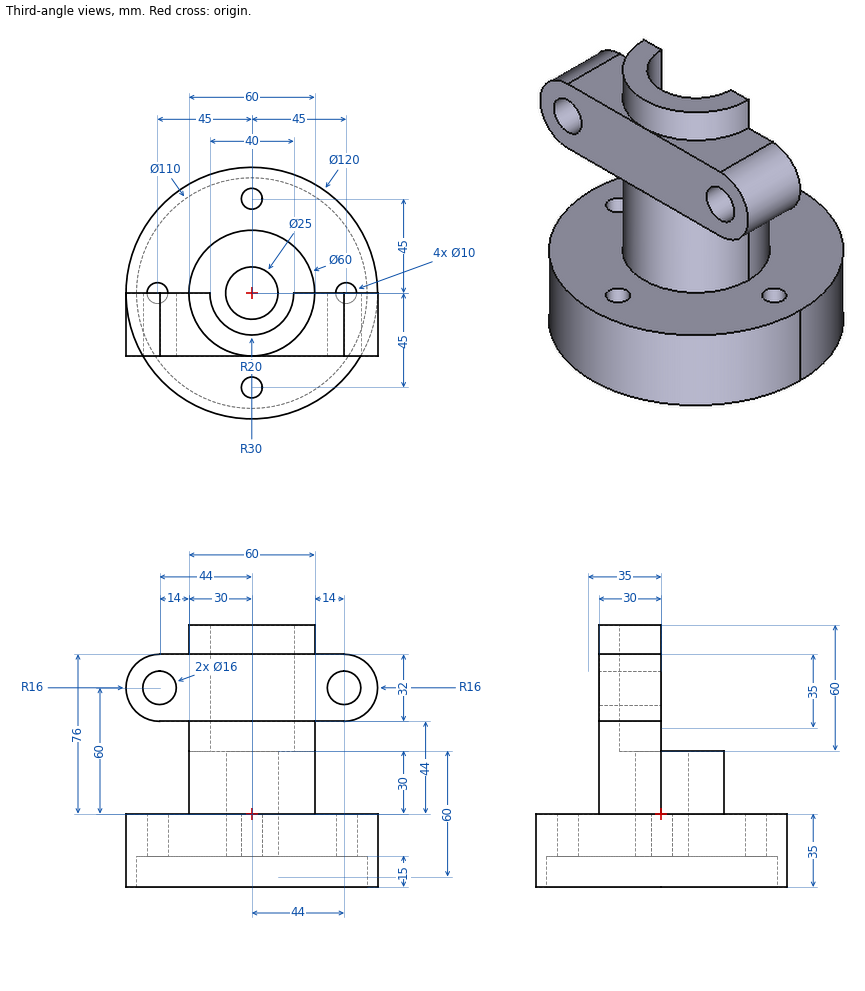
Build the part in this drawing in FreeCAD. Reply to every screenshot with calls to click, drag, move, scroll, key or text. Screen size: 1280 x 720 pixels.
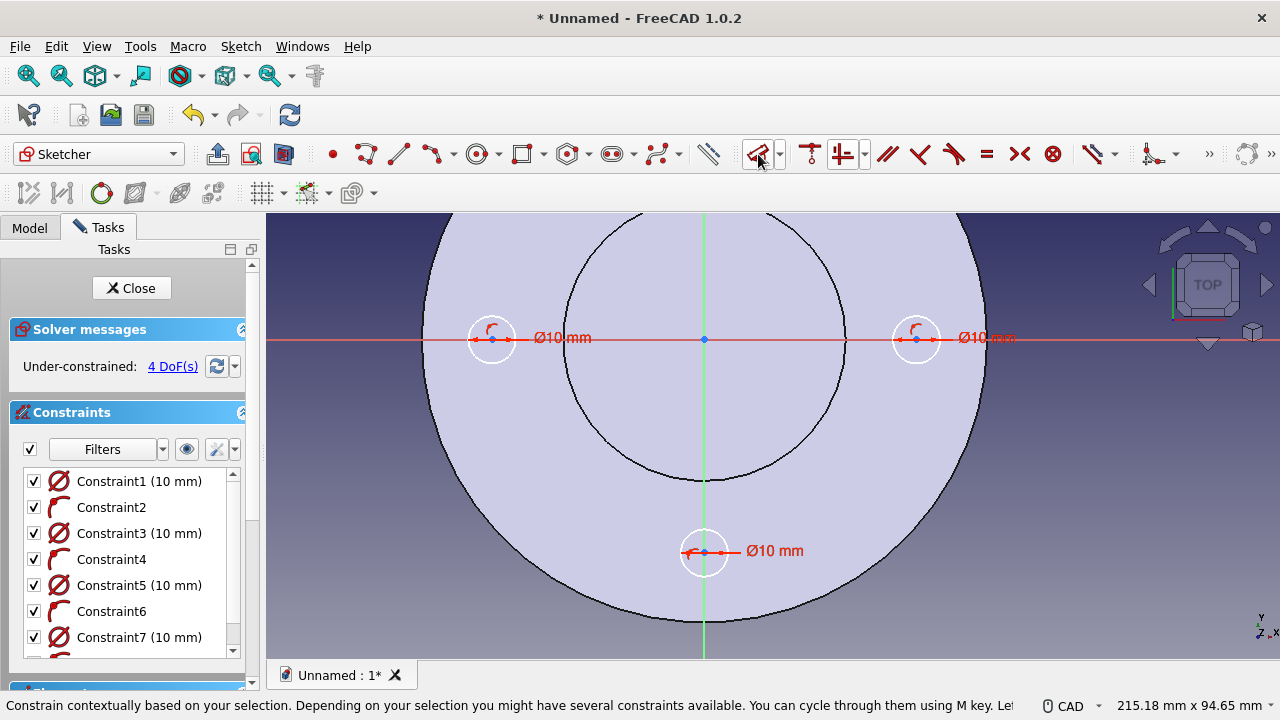
click(917, 340)
click(810, 374)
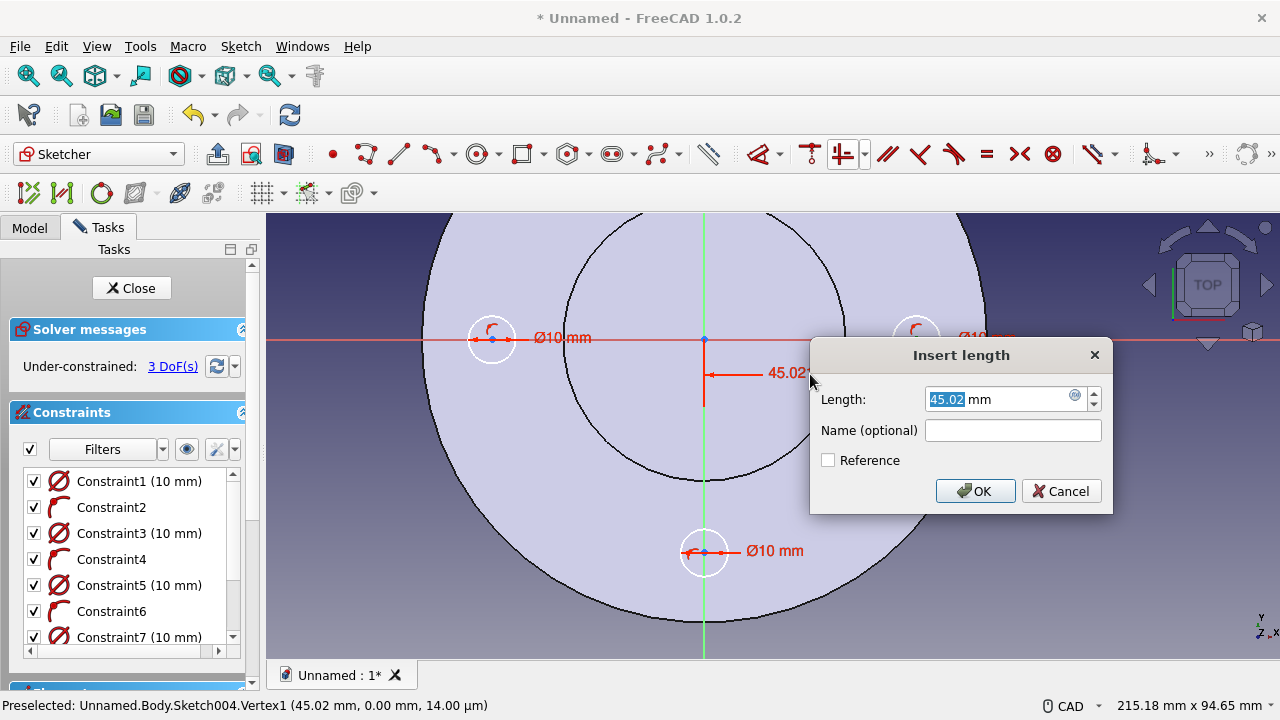
text(45)
key(Return)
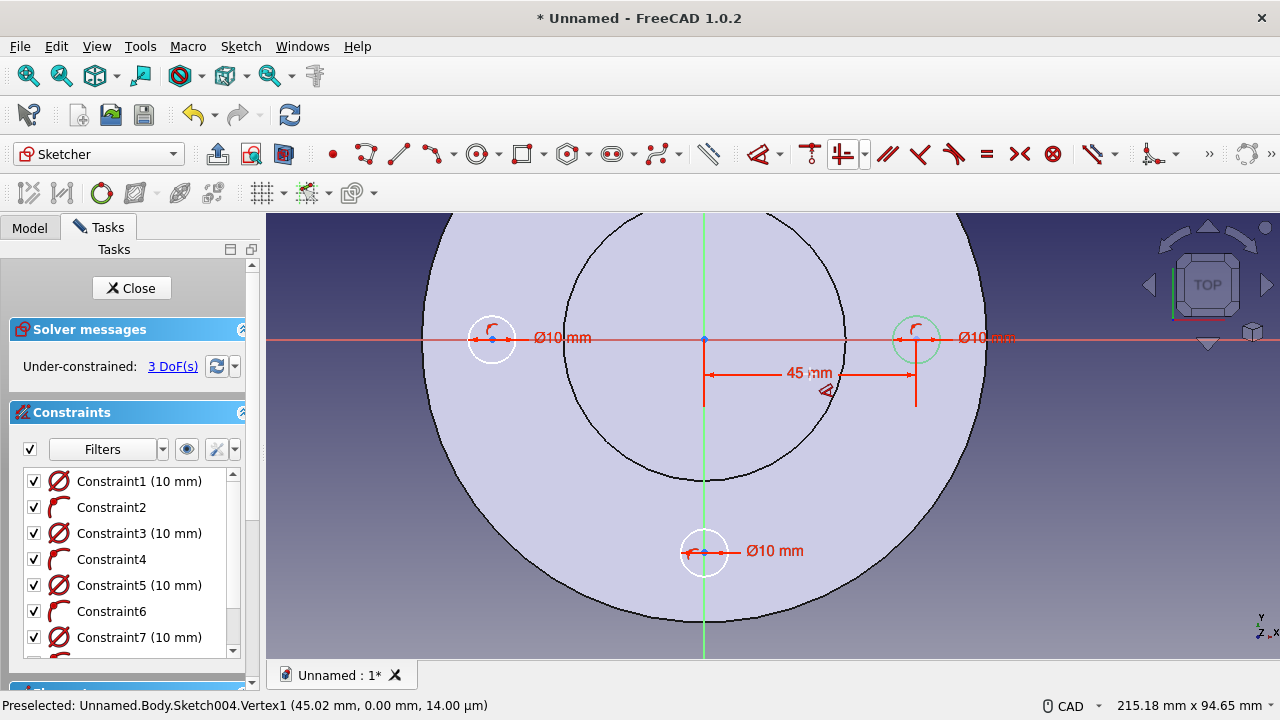
scroll(705, 553, down, 3)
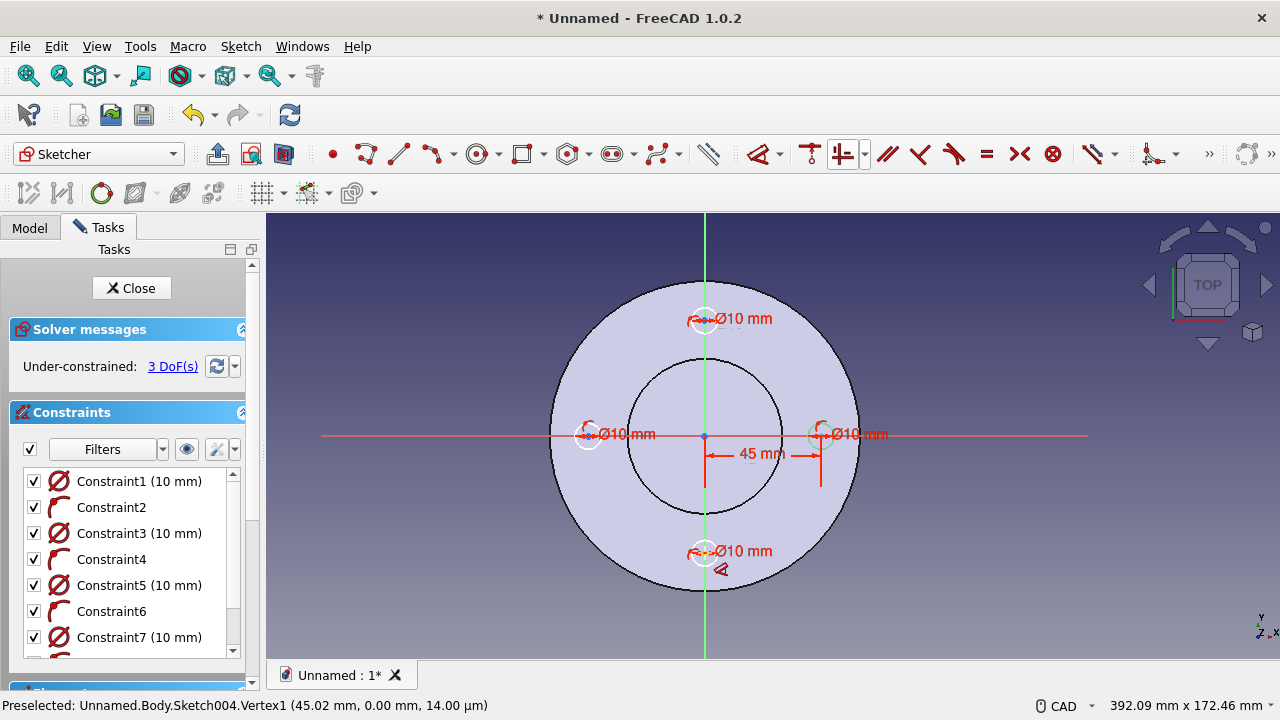
click(705, 321)
click(739, 378)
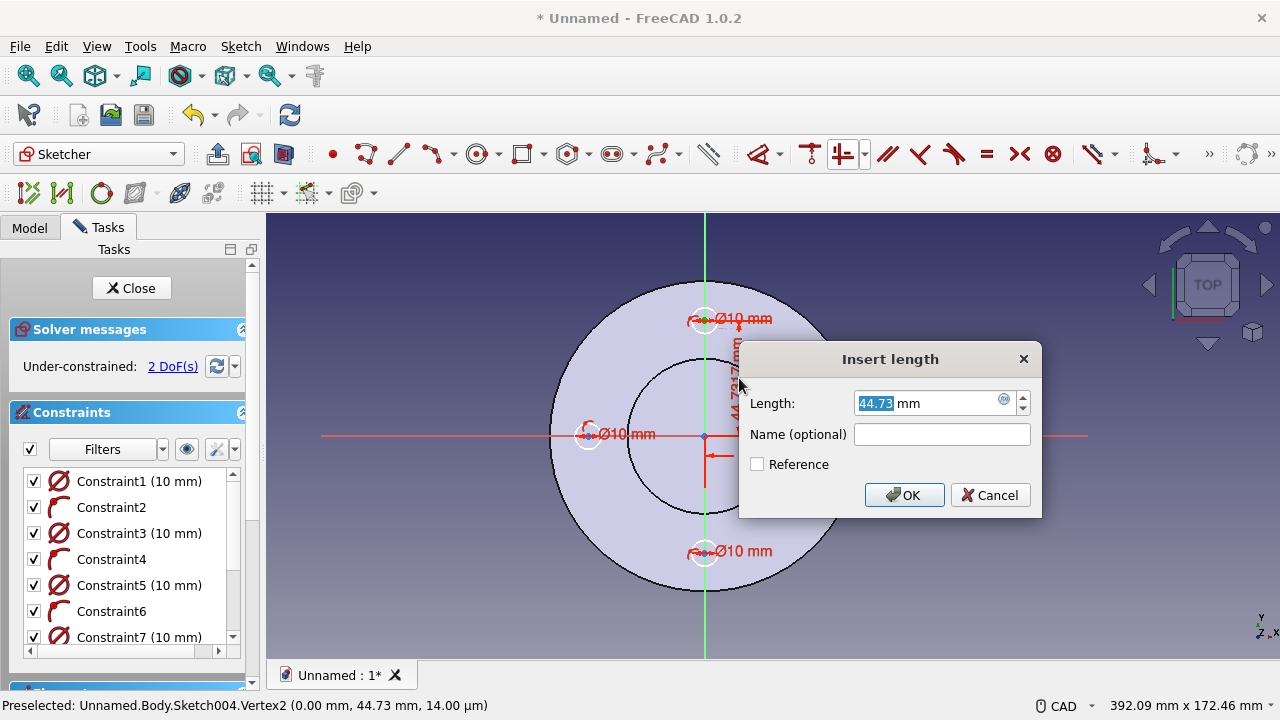
text(45)
key(Return)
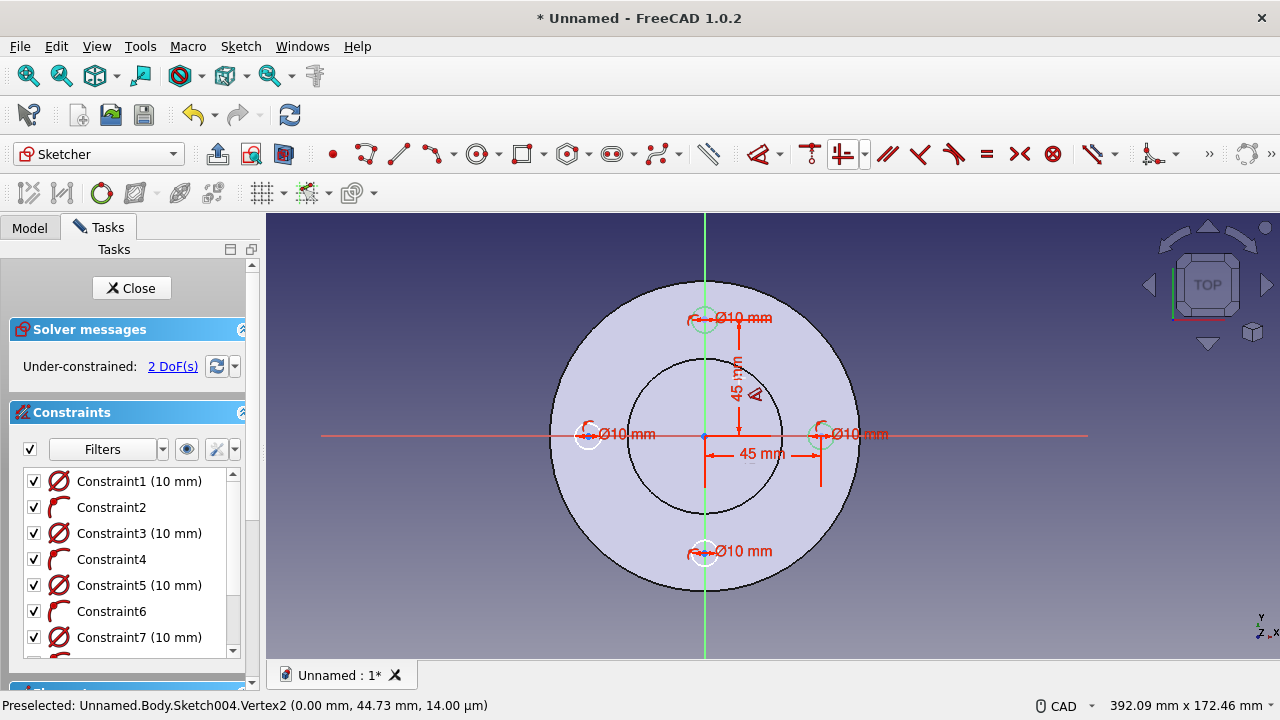
click(588, 436)
click(647, 470)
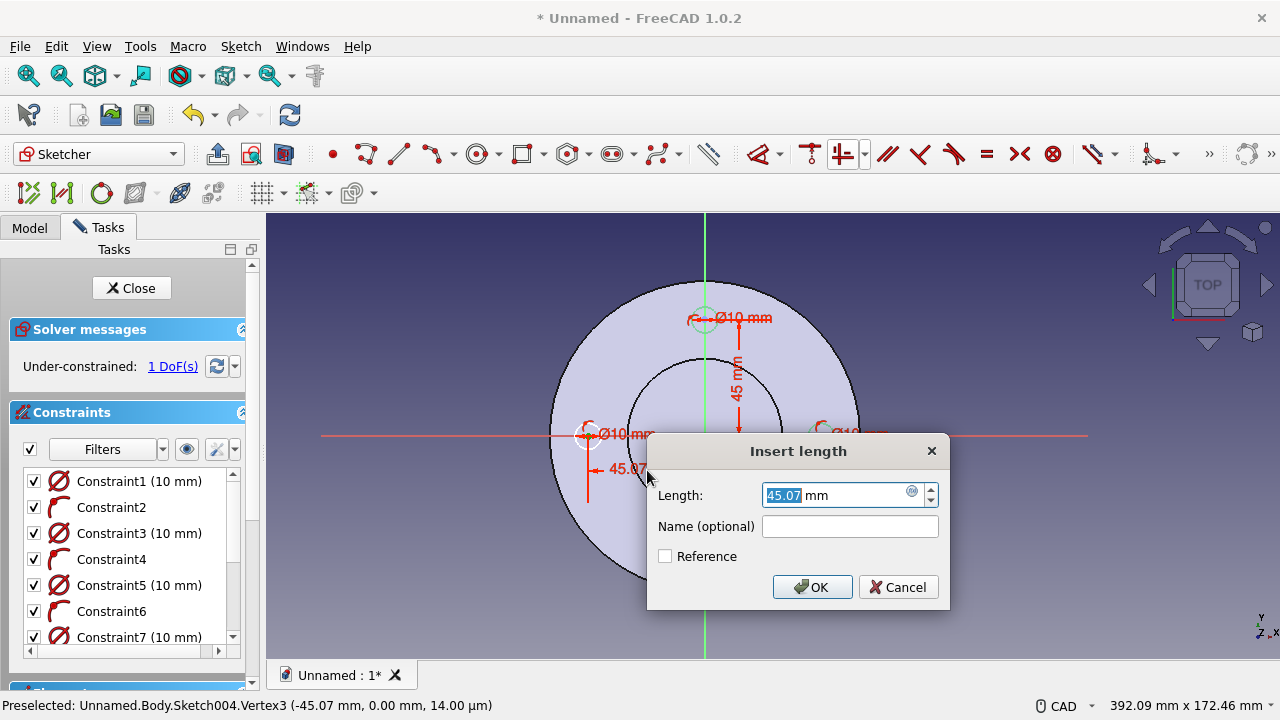
text(45)
key(Return)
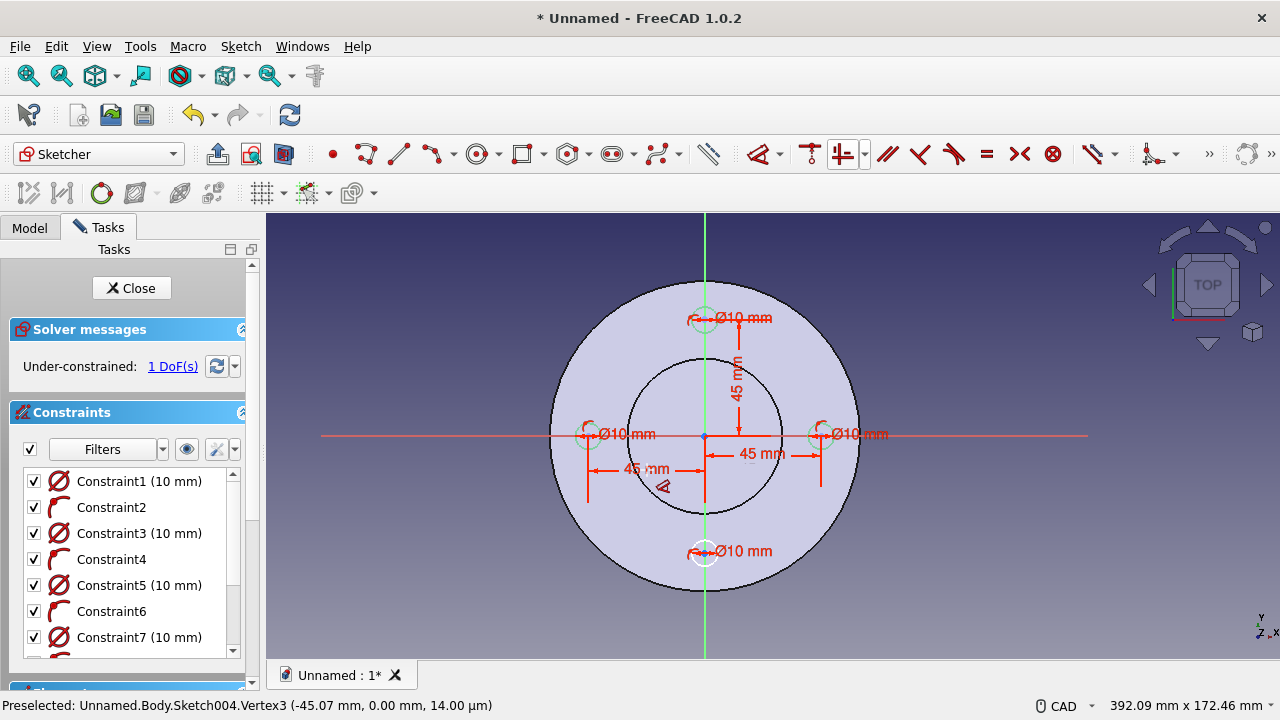
click(705, 553)
click(739, 495)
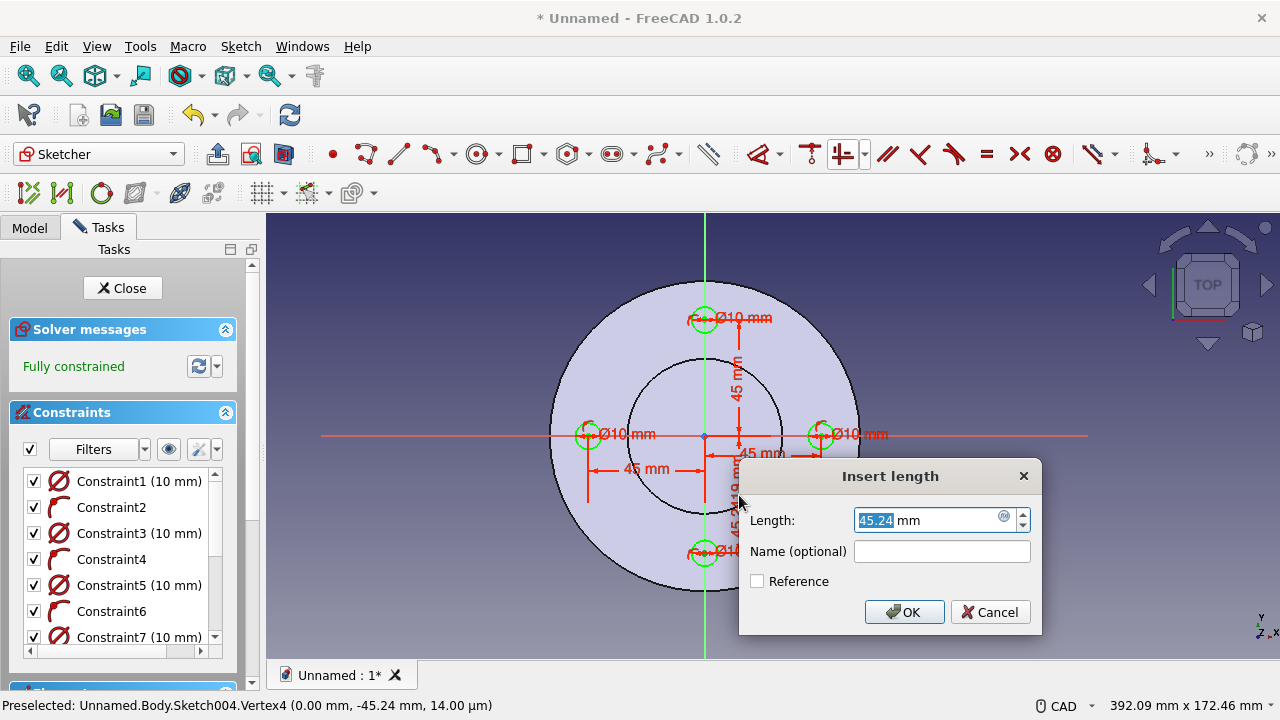
text(45)
key(Return)
key(Escape)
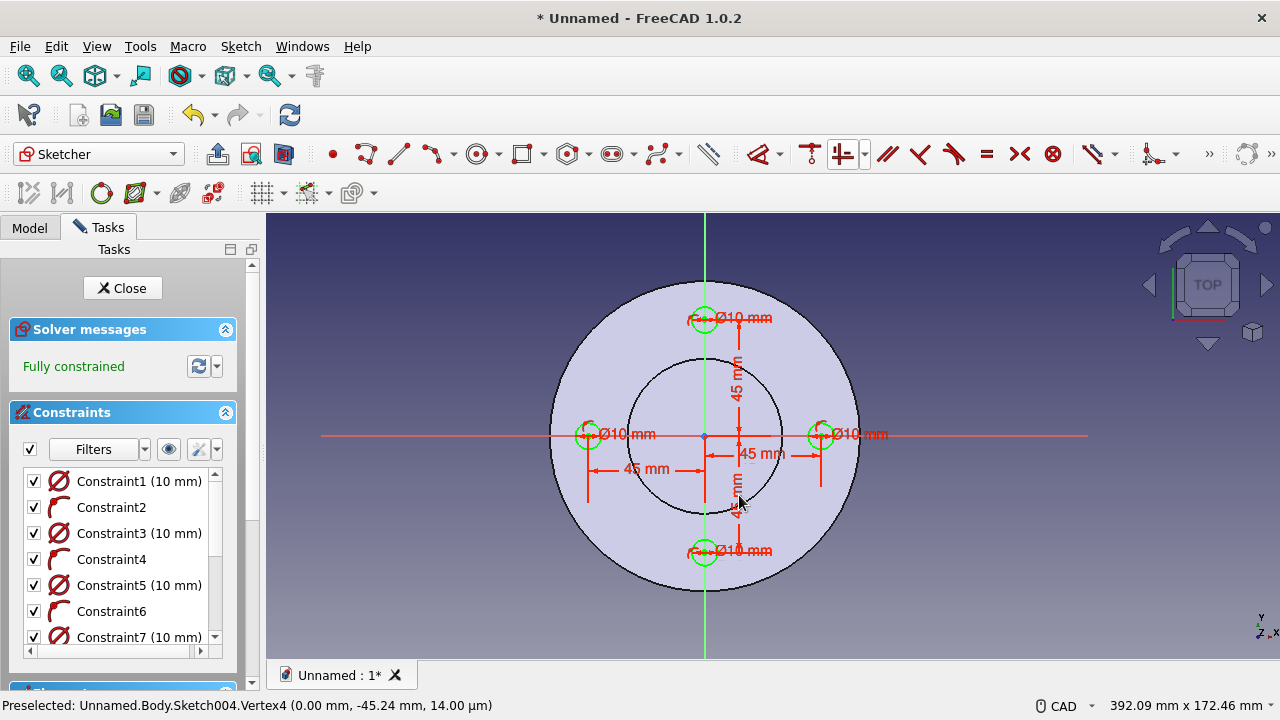
click(123, 288)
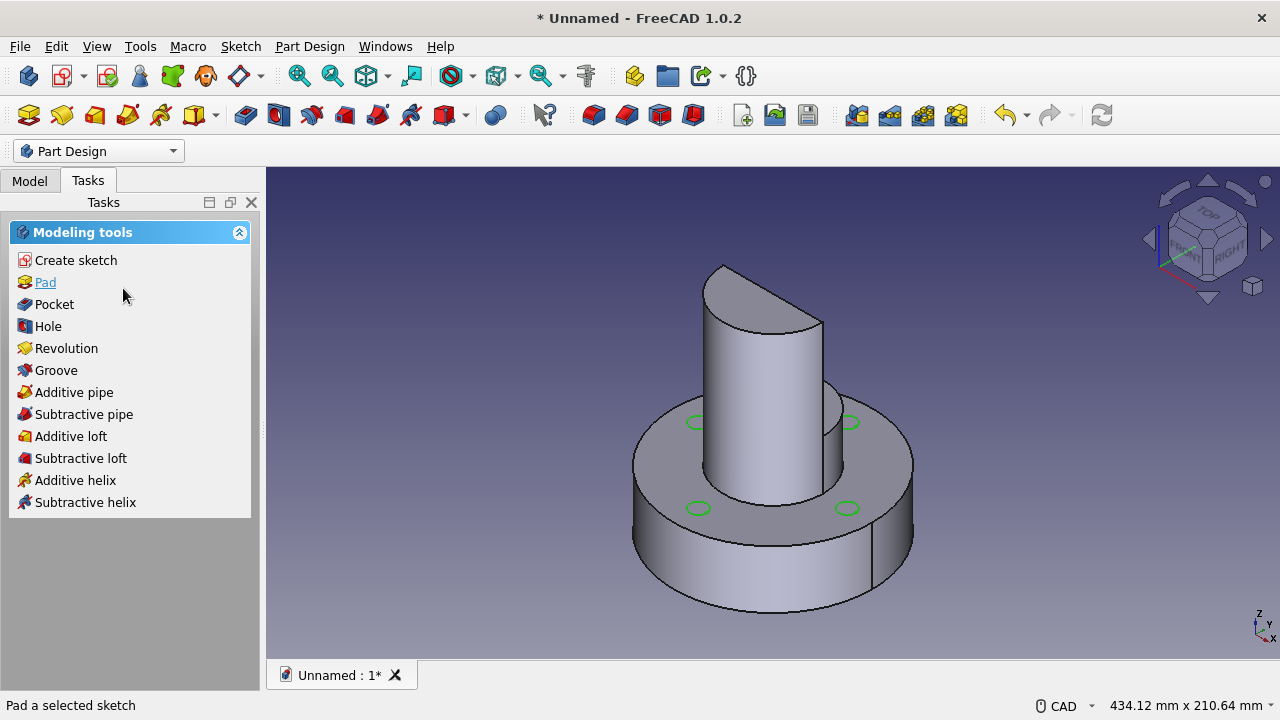
click(246, 116)